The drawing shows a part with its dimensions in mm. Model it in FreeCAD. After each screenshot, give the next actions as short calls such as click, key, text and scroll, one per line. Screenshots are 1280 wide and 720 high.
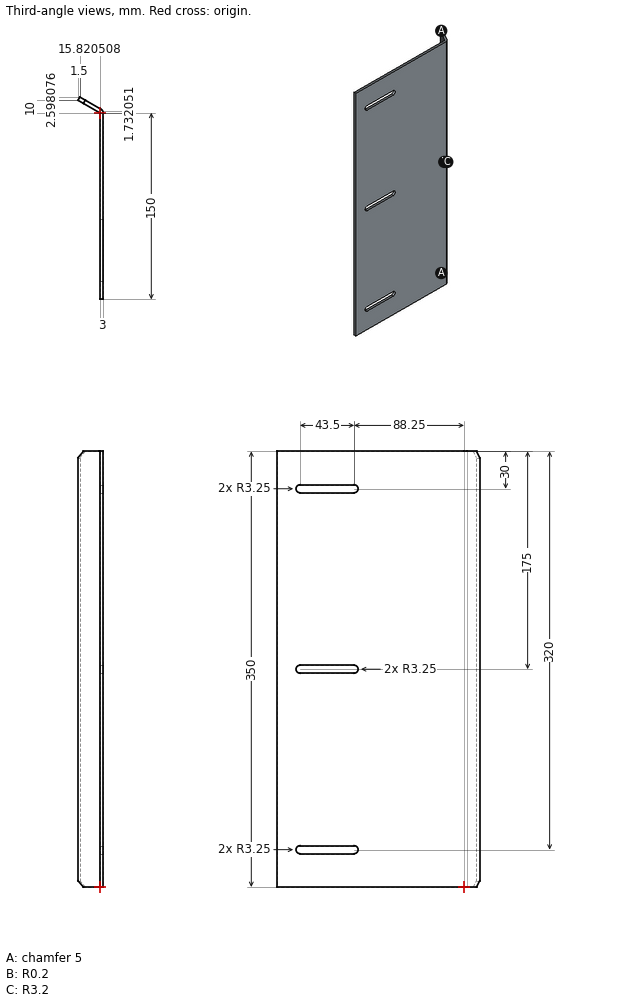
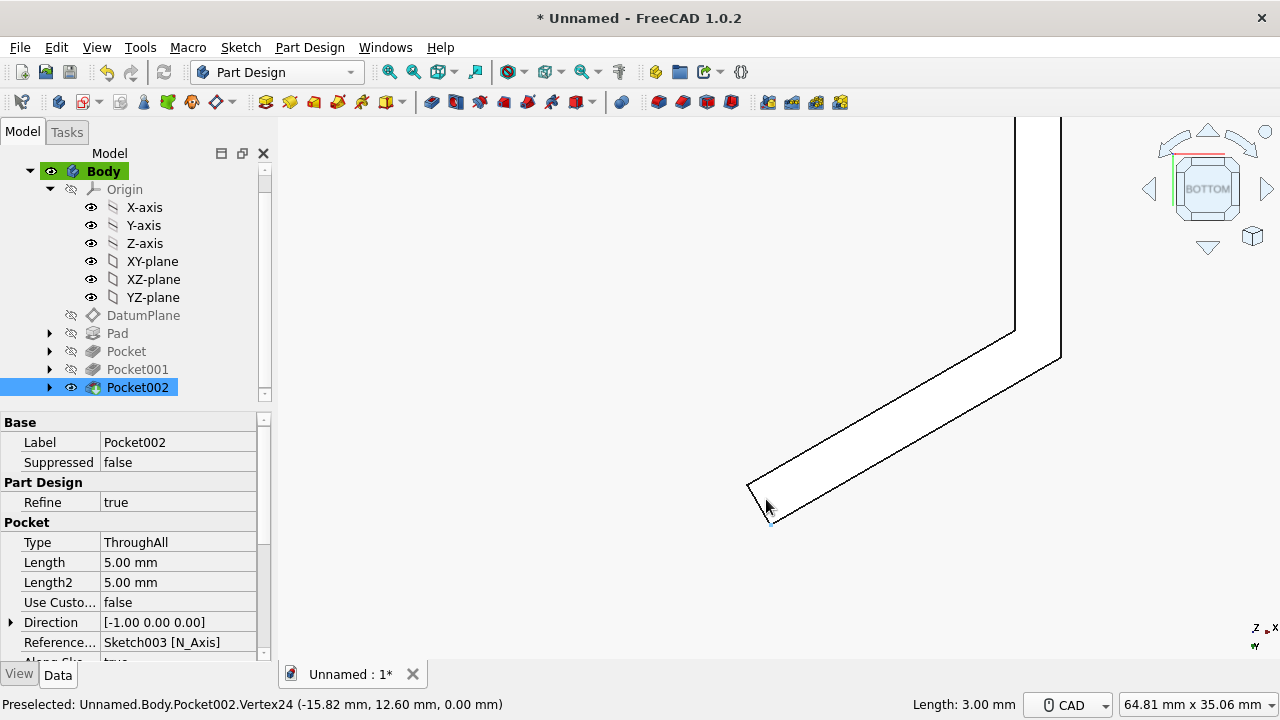
click(759, 504, ctrl)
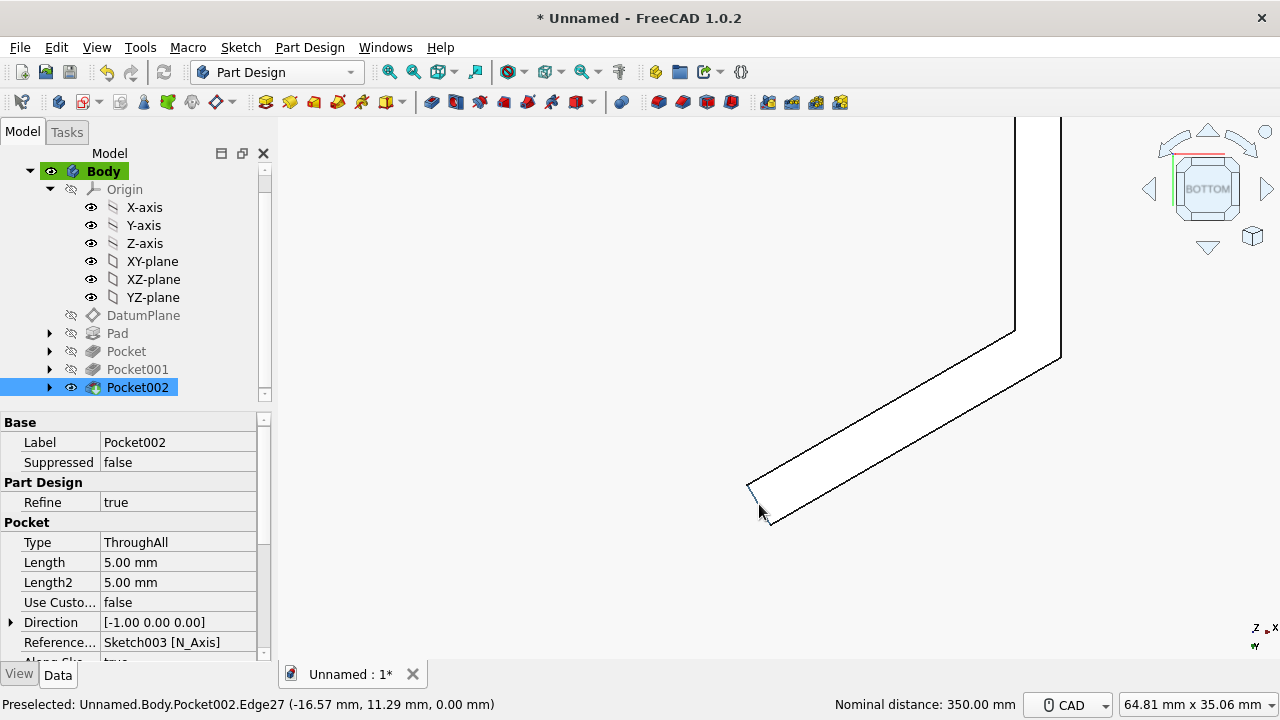
click(684, 102)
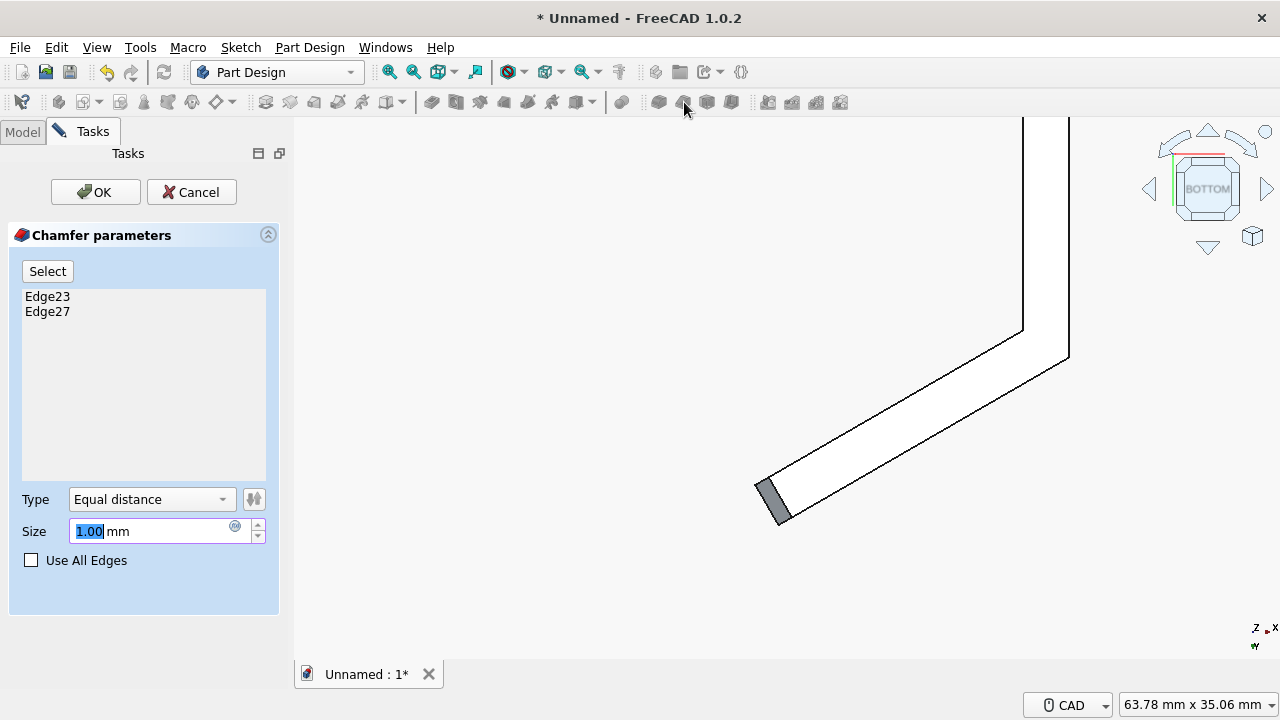
text(5)
key(Tab)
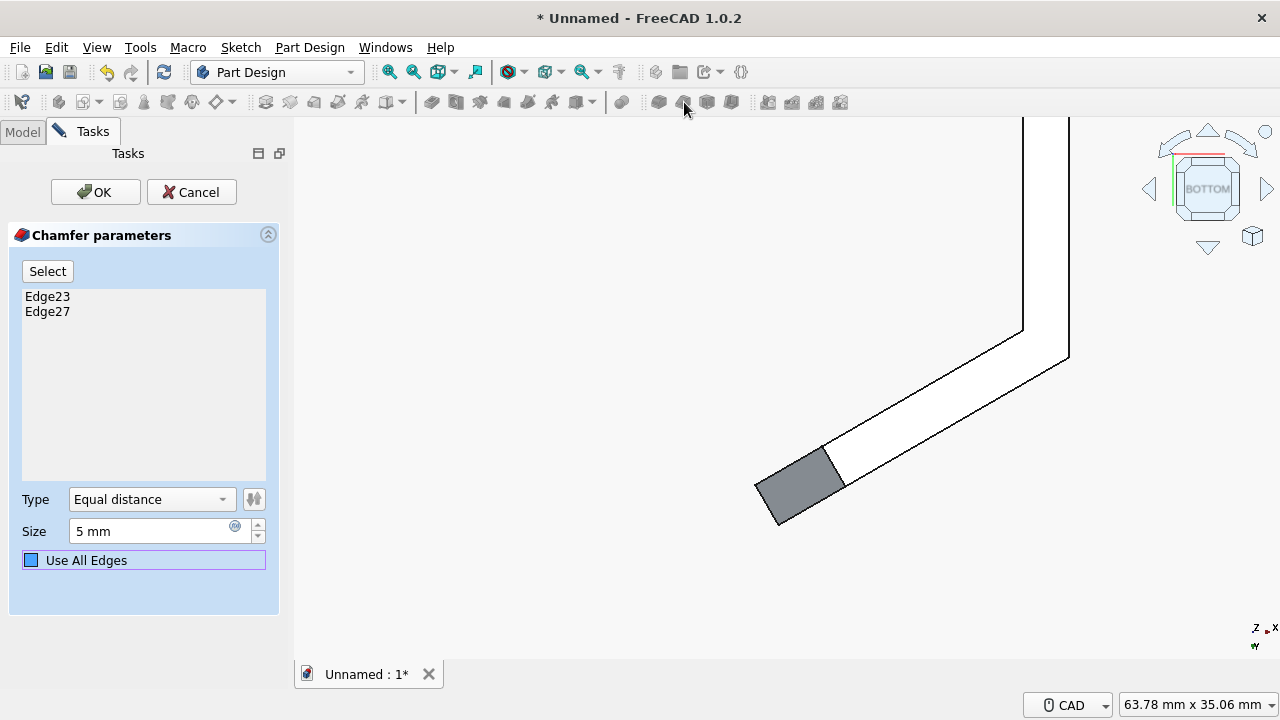
click(96, 192)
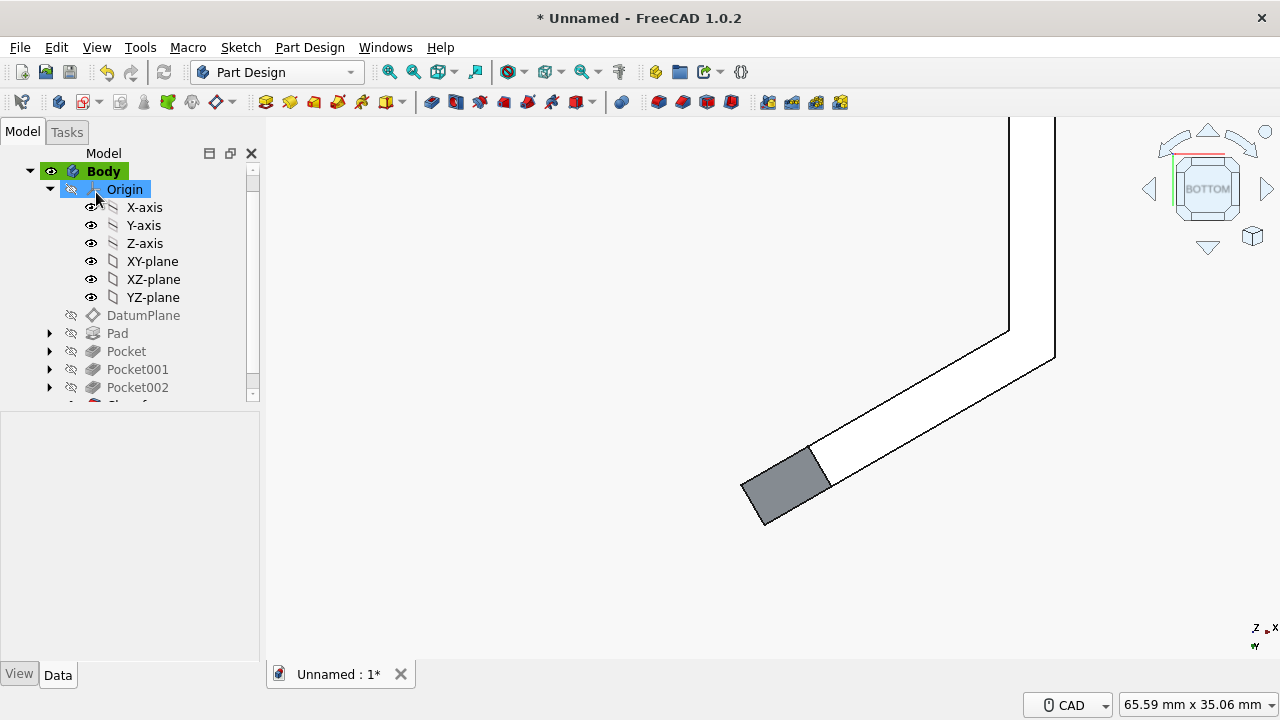
click(390, 72)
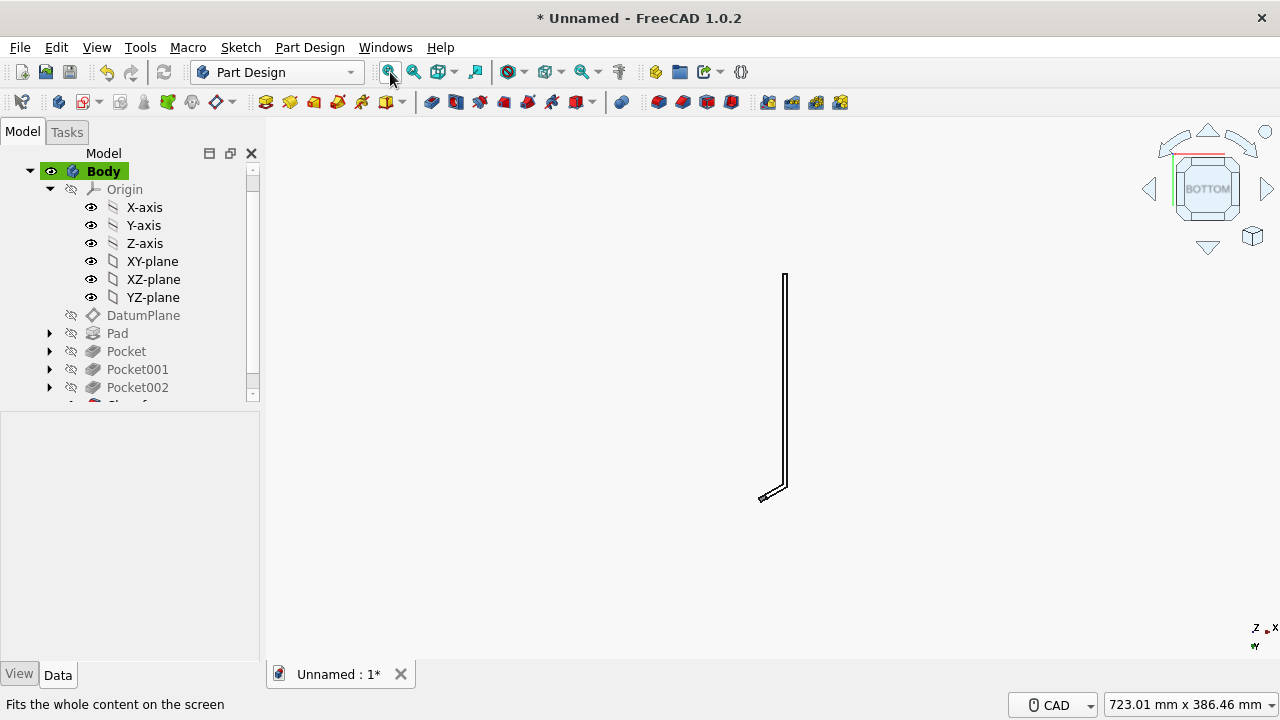
key(0)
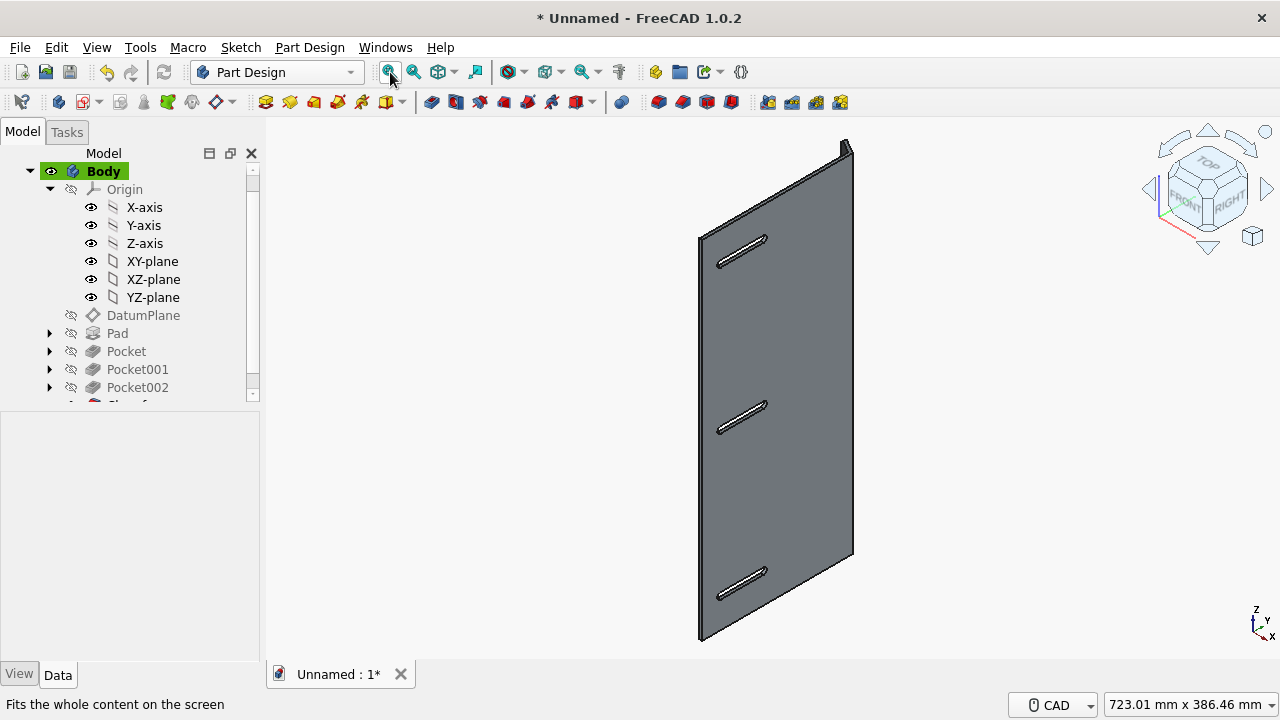
key(2)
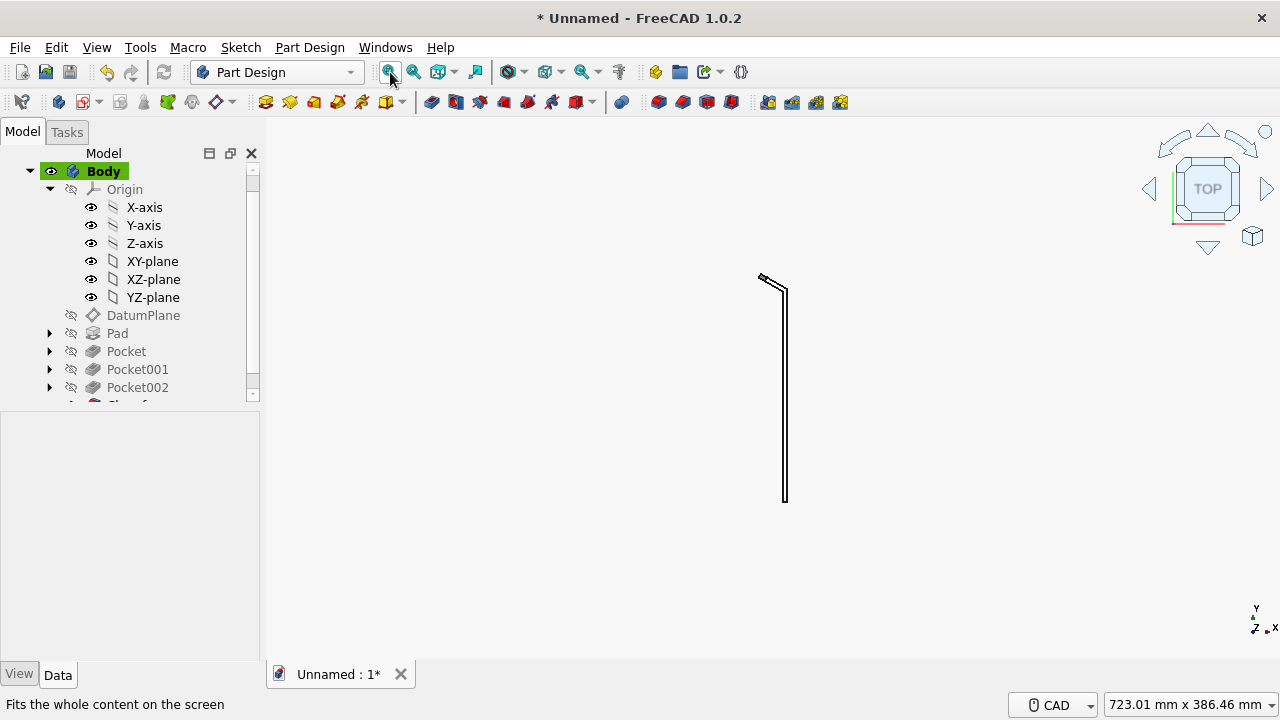
click(390, 72)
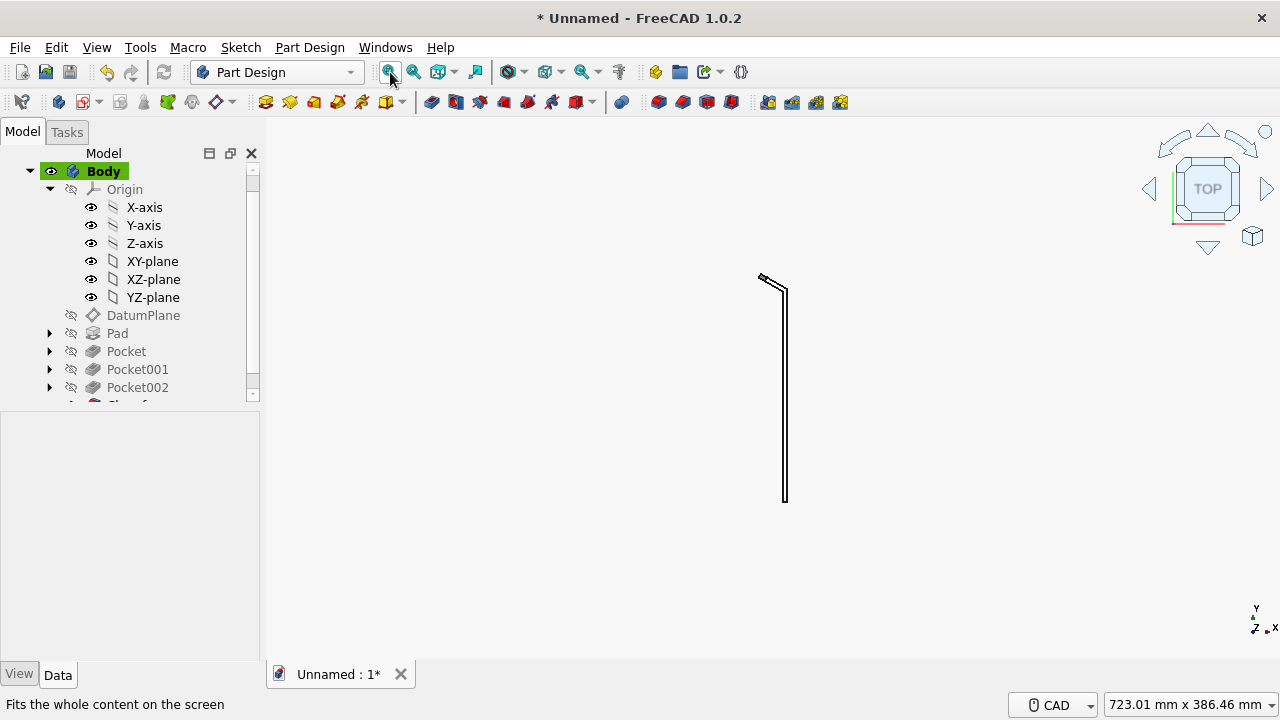
key(1)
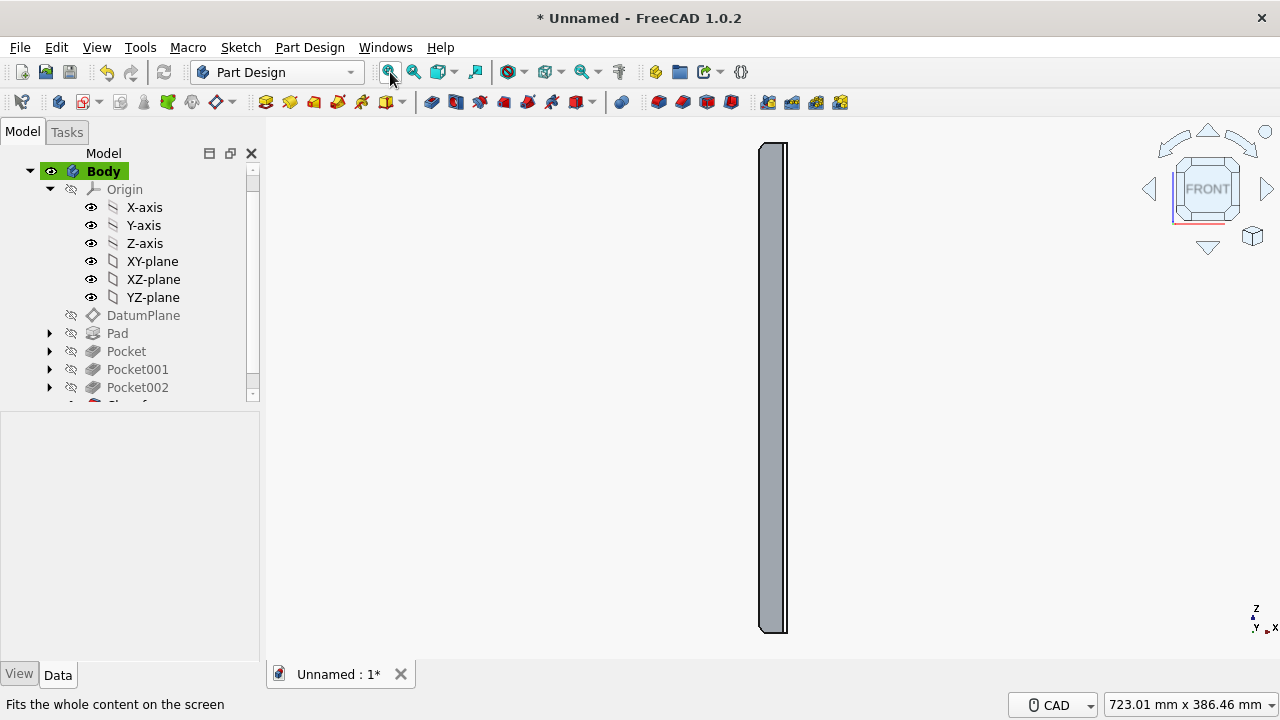
key(3)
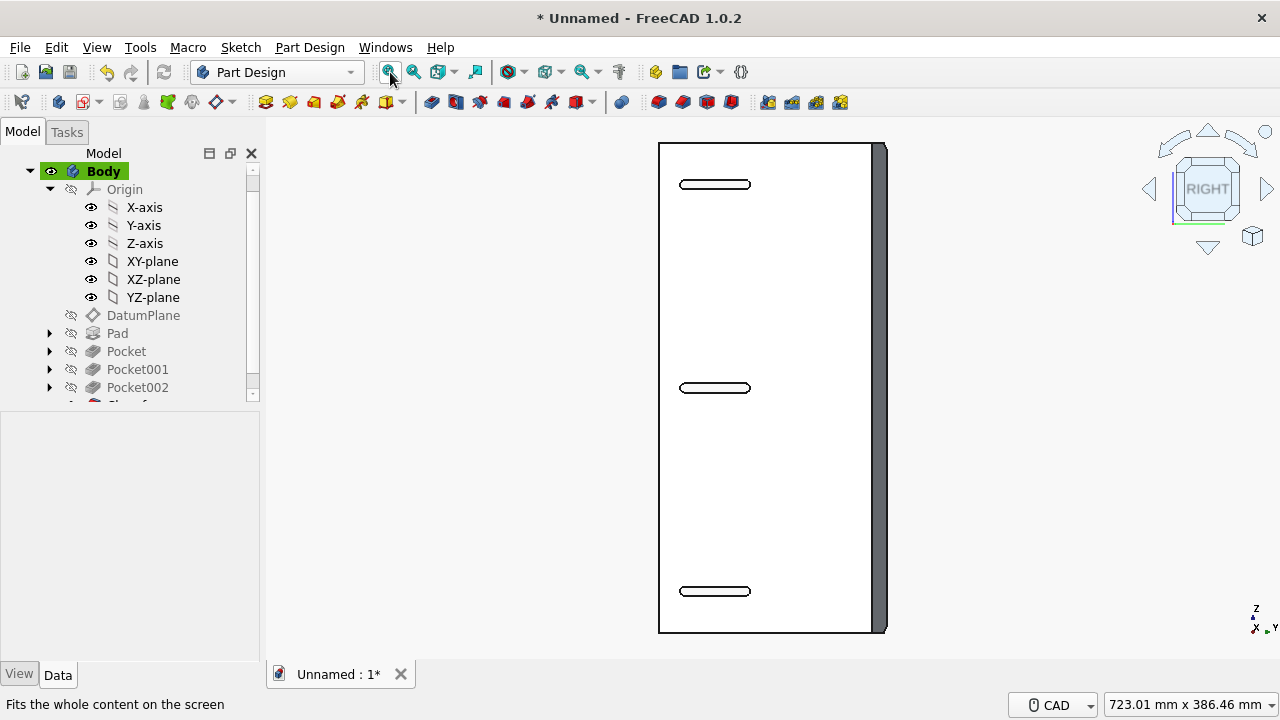
key(5)